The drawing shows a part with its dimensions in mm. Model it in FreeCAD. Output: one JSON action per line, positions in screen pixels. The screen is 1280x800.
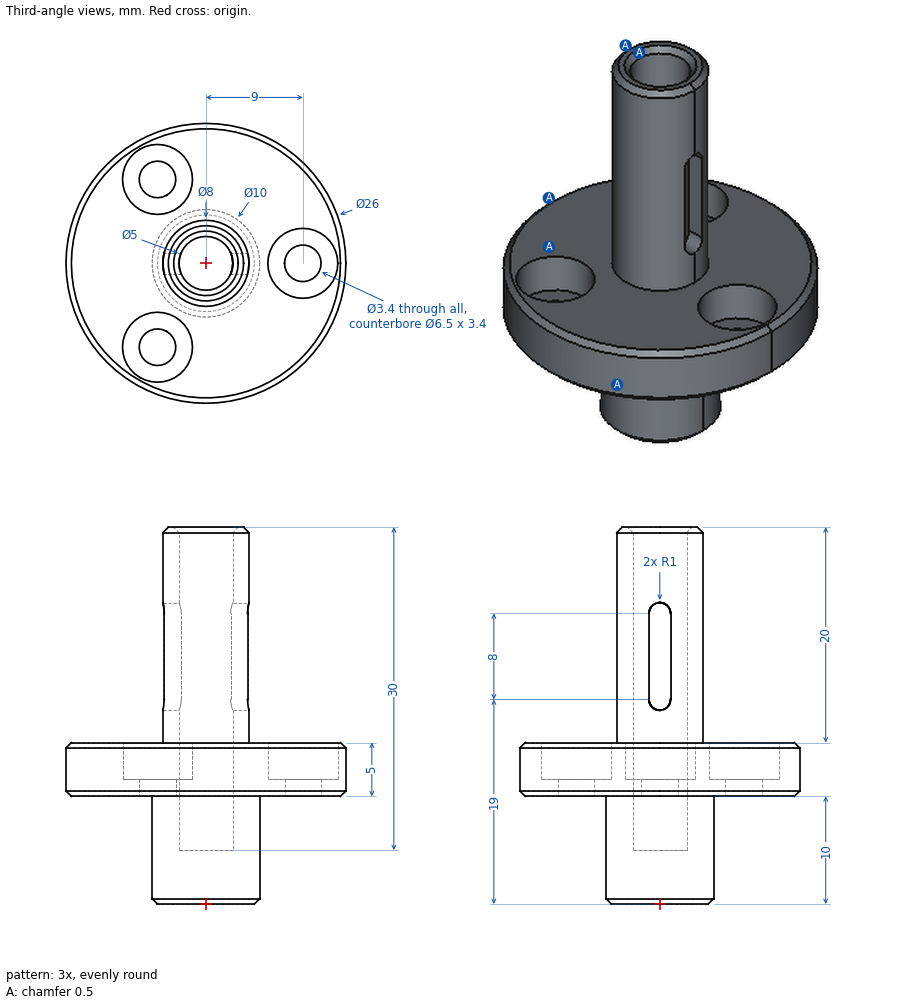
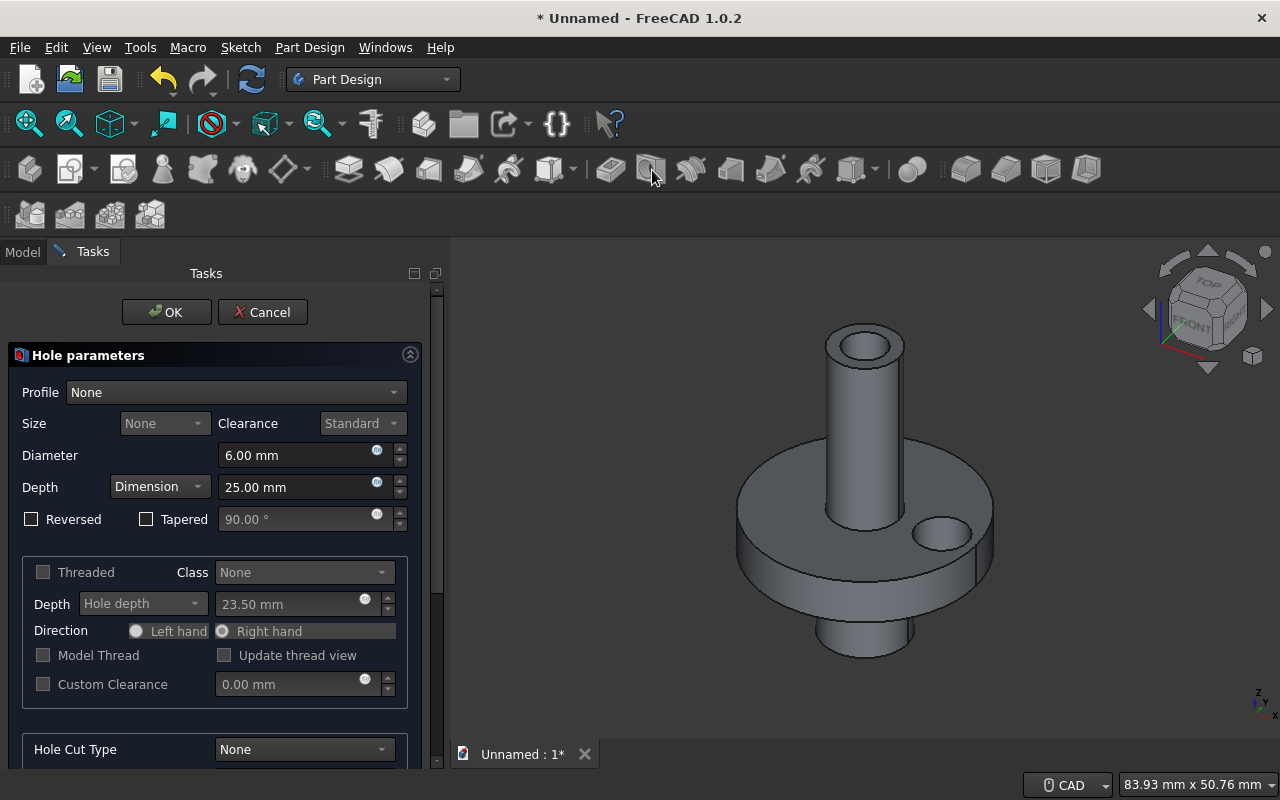
{"action": "triple_click", "coordinate": [305, 455]}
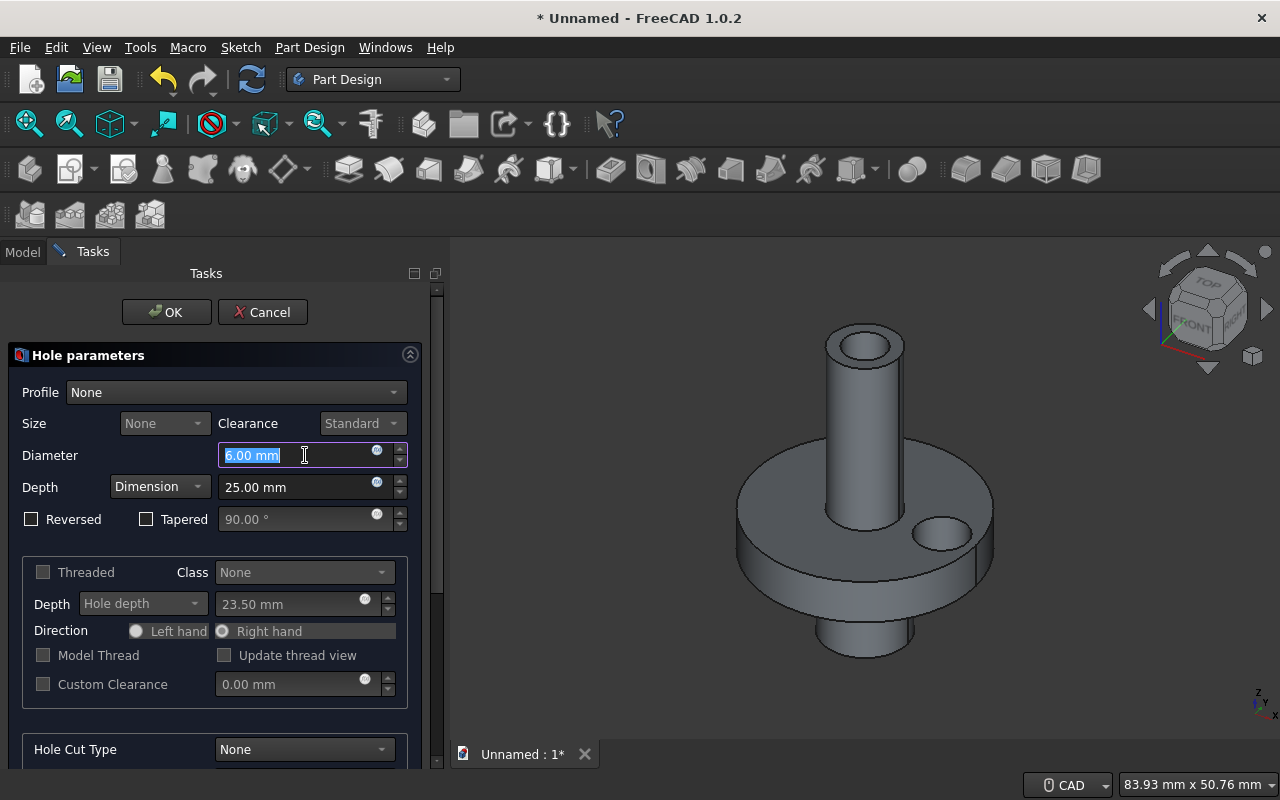
{"action": "type", "text": "3.4"}
{"action": "key", "text": "Tab"}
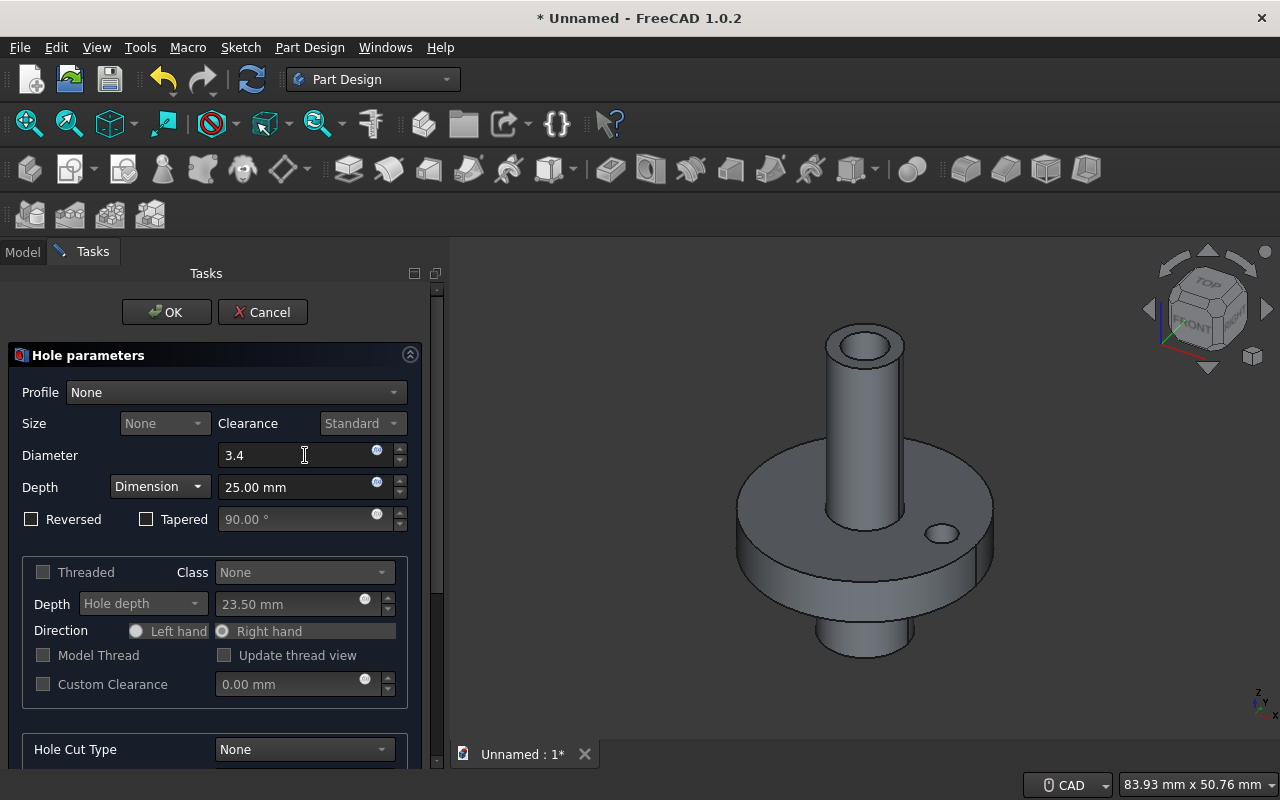
{"action": "left_click", "coordinate": [161, 486]}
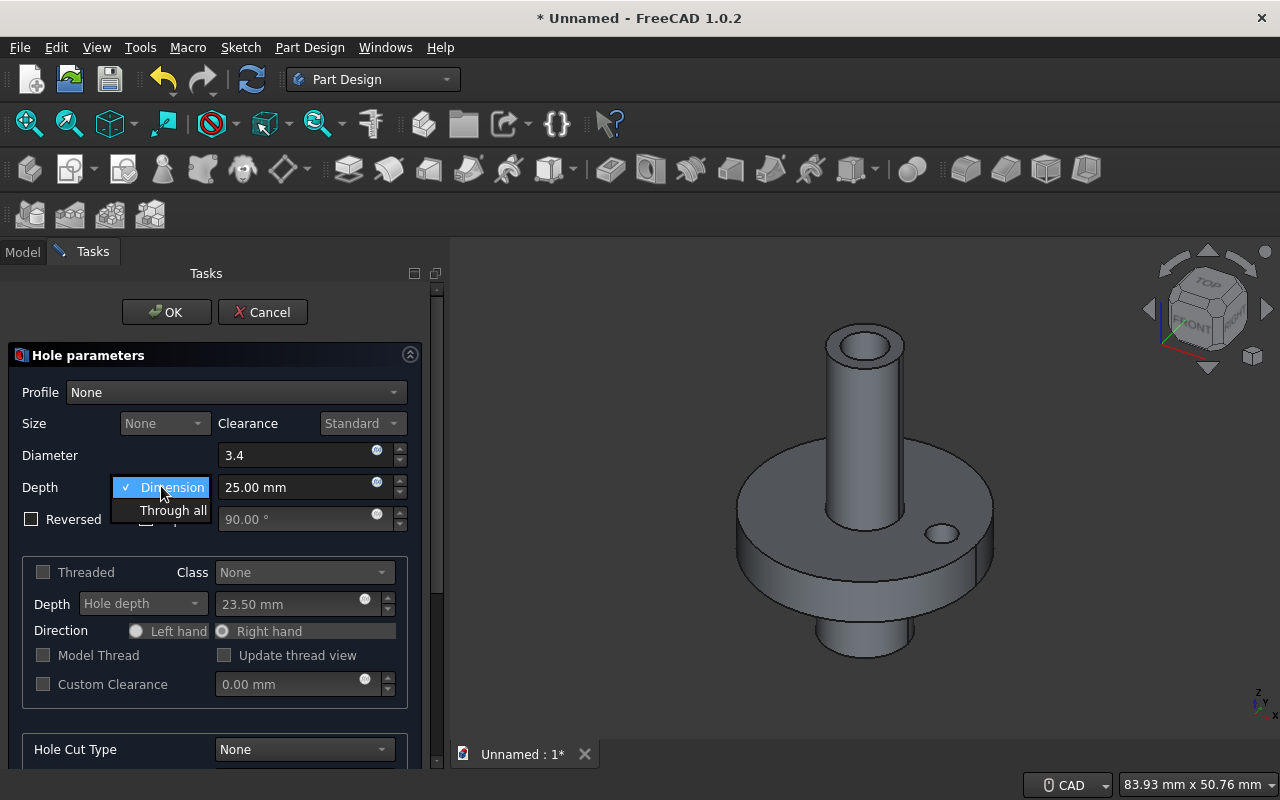
{"action": "left_click", "coordinate": [160, 510]}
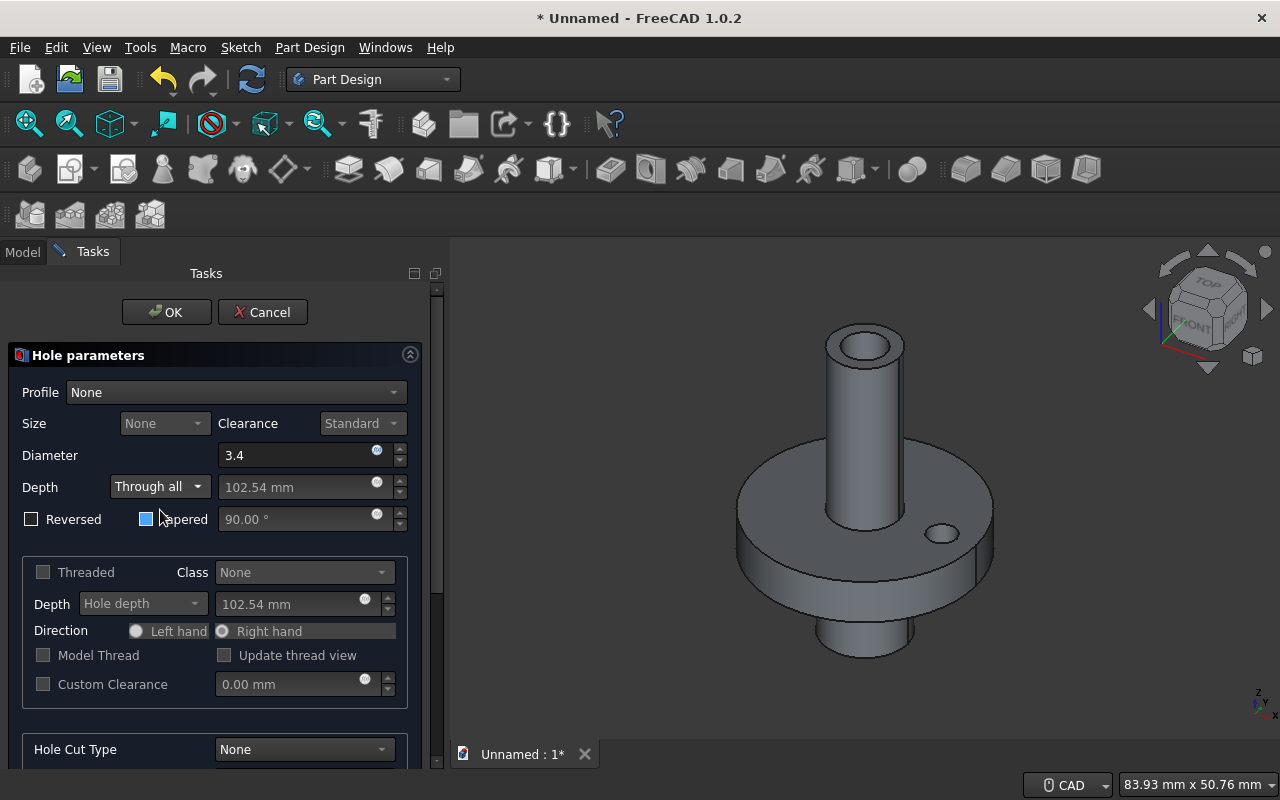
{"action": "left_click", "coordinate": [306, 750]}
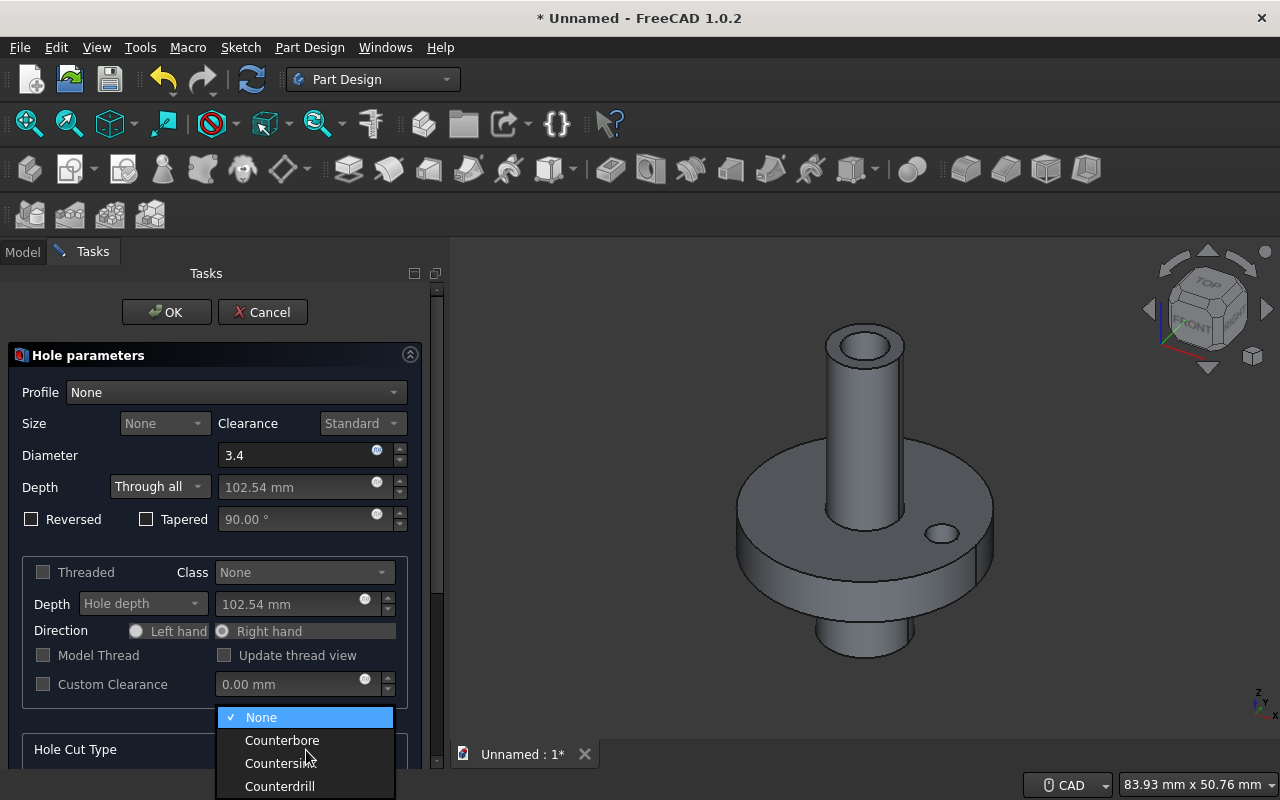
{"action": "left_click", "coordinate": [304, 740]}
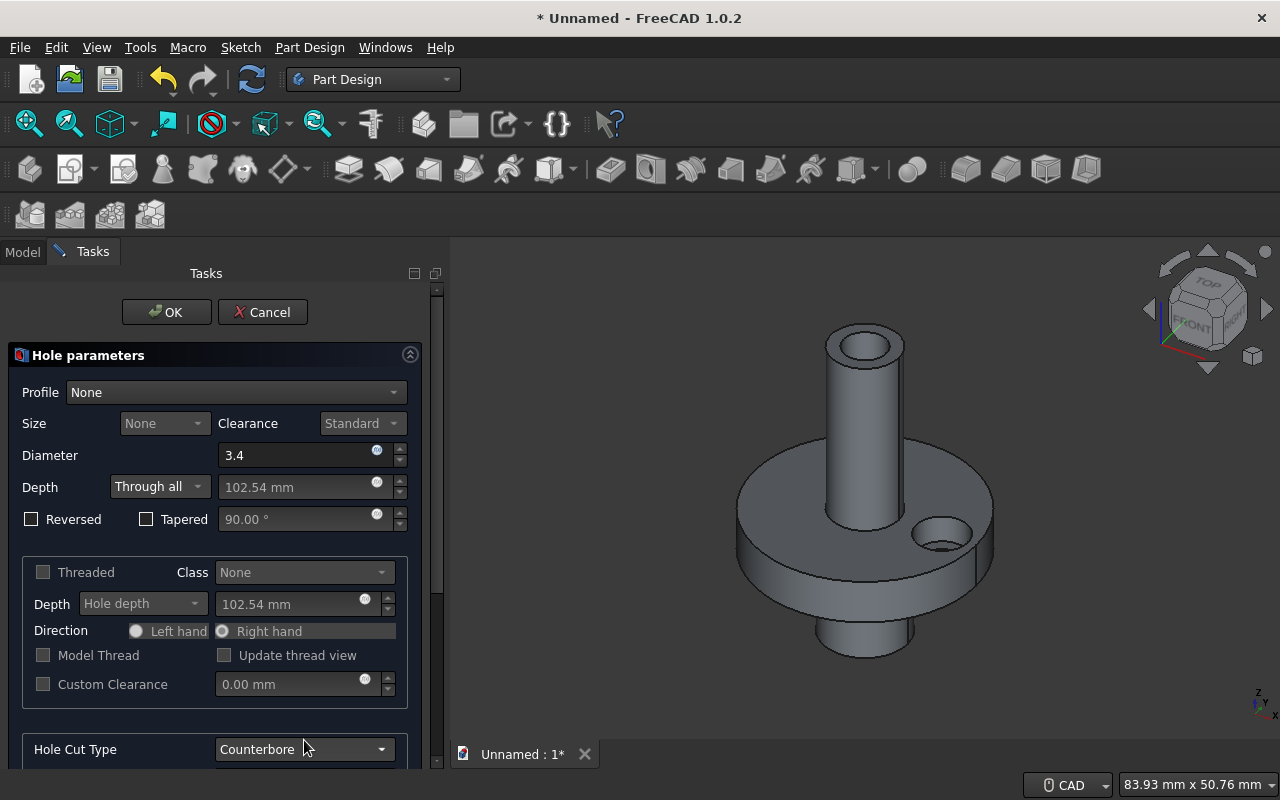
{"action": "scroll", "coordinate": [437, 526], "scroll_direction": "down", "scroll_amount": 2}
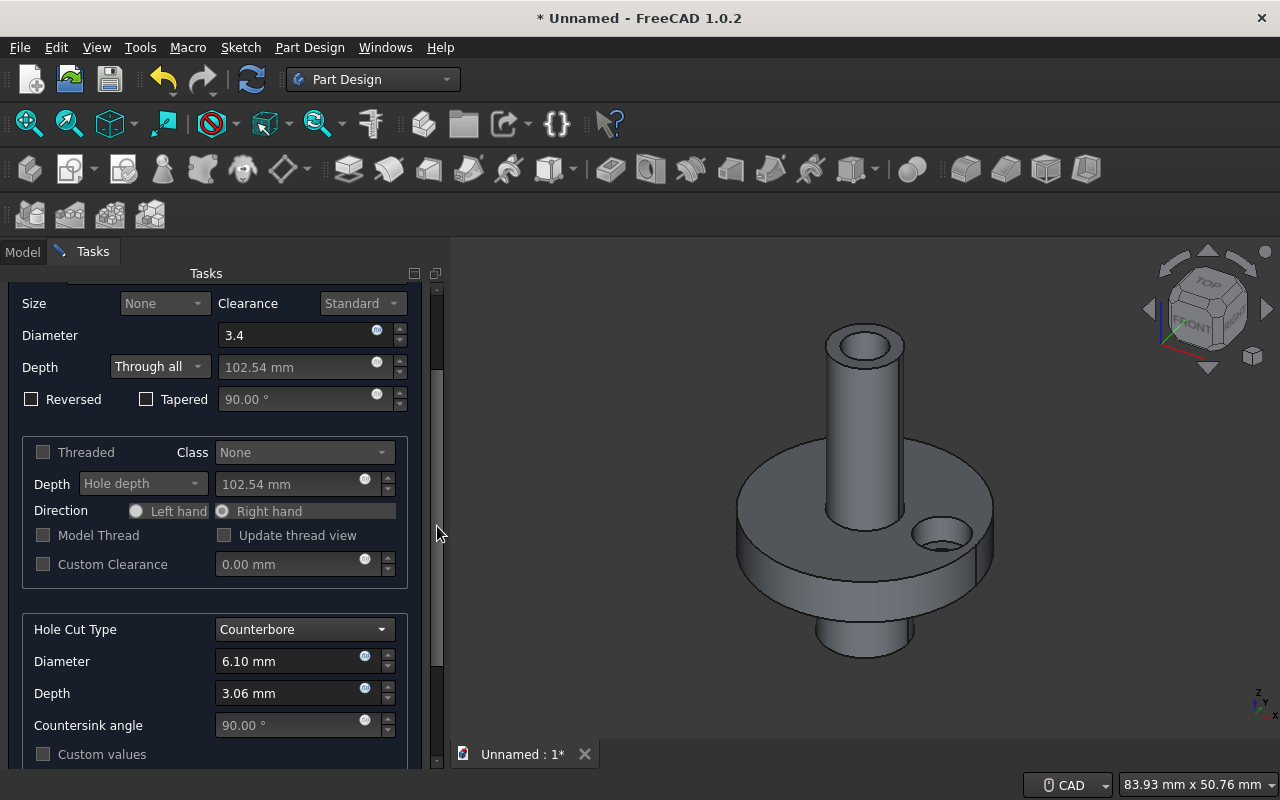
{"action": "triple_click", "coordinate": [298, 661]}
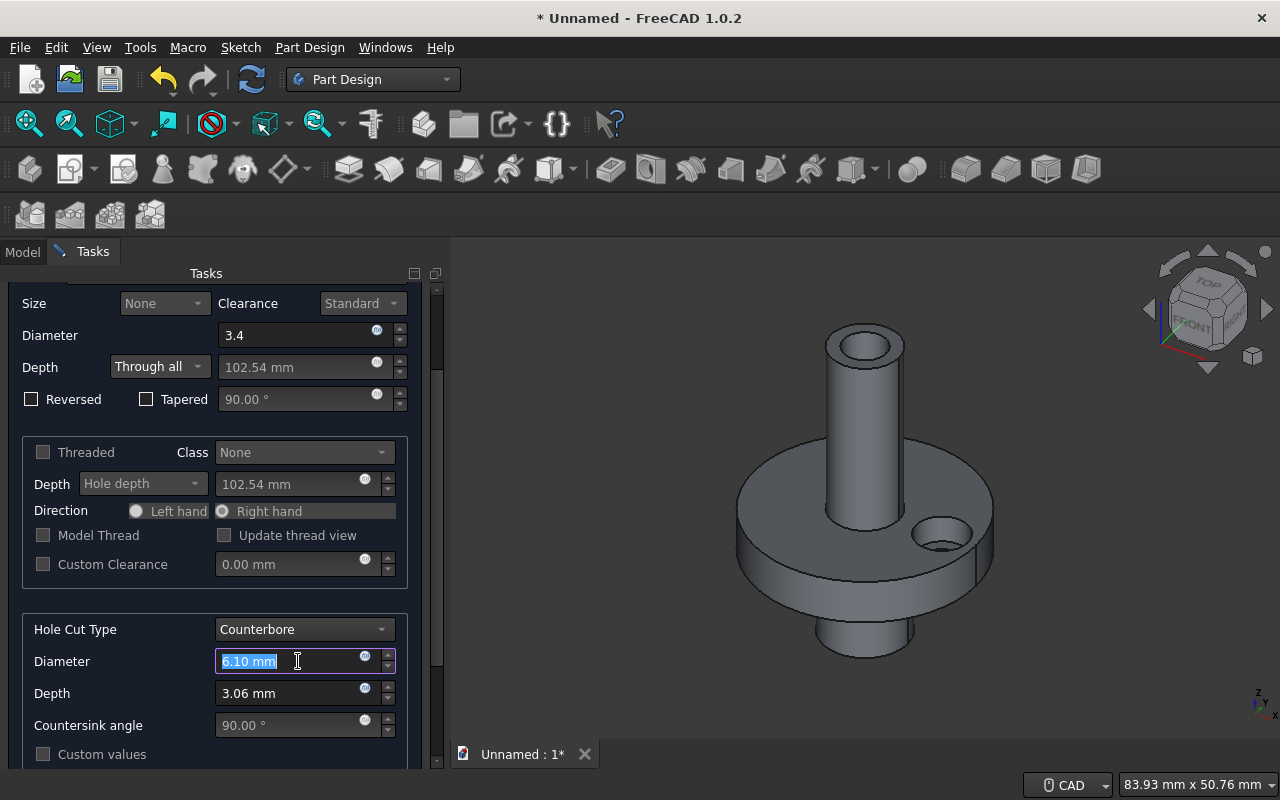
{"action": "type", "text": "6.5"}
{"action": "key", "text": "Tab"}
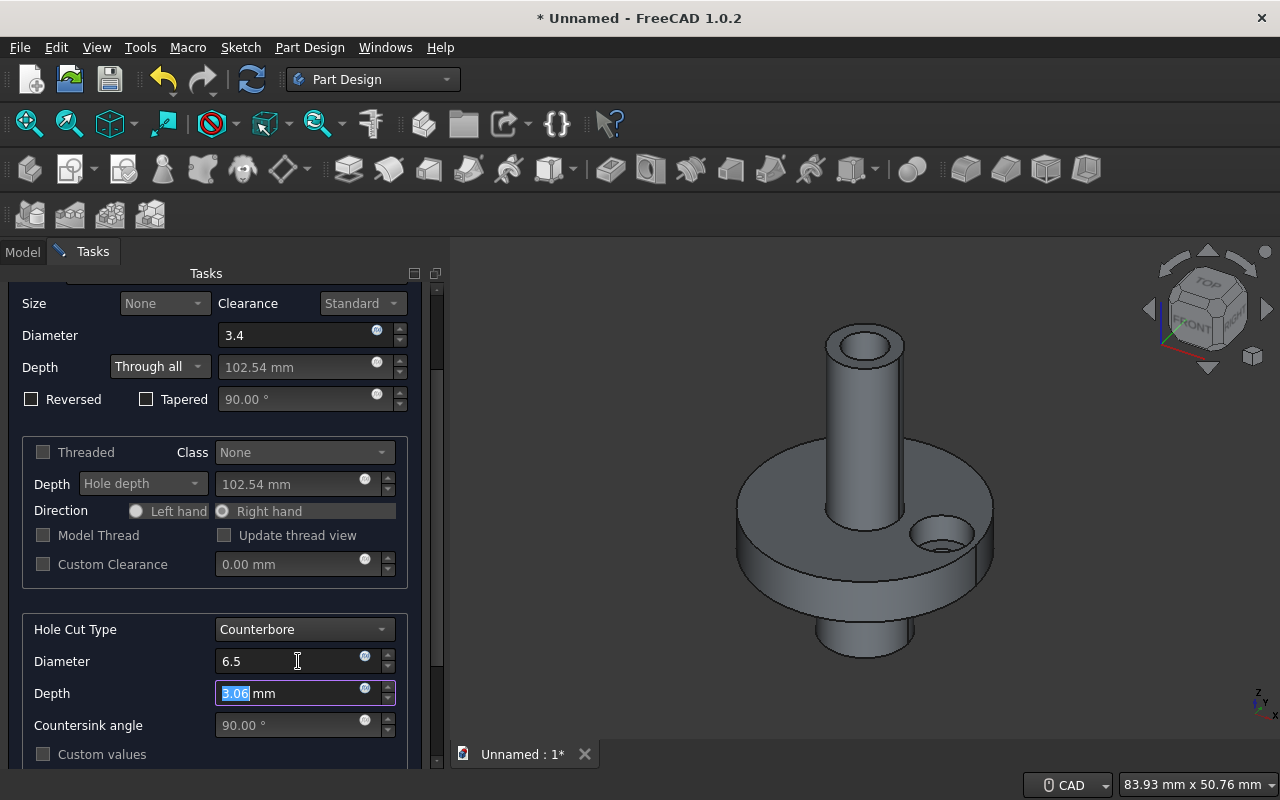
{"action": "type", "text": "3.4"}
{"action": "key", "text": "Tab"}